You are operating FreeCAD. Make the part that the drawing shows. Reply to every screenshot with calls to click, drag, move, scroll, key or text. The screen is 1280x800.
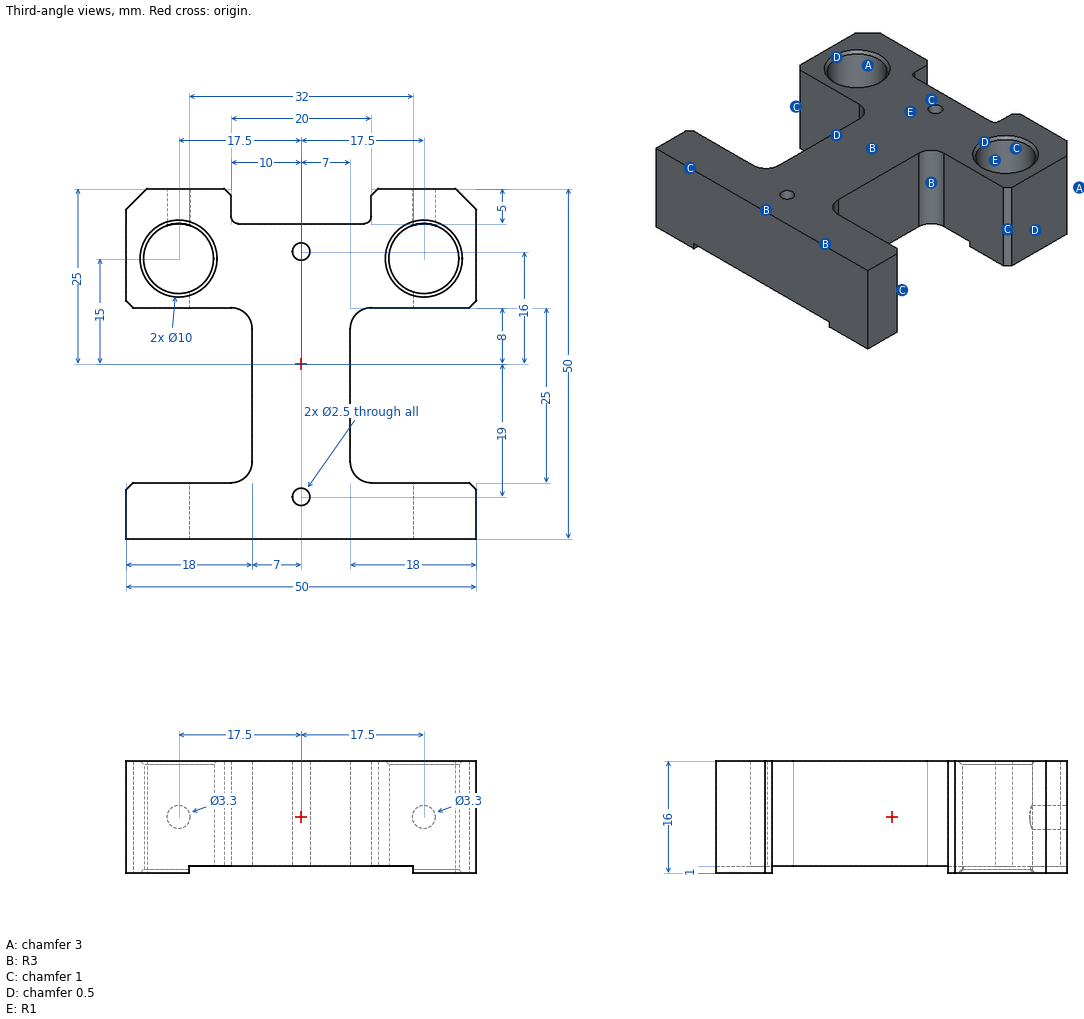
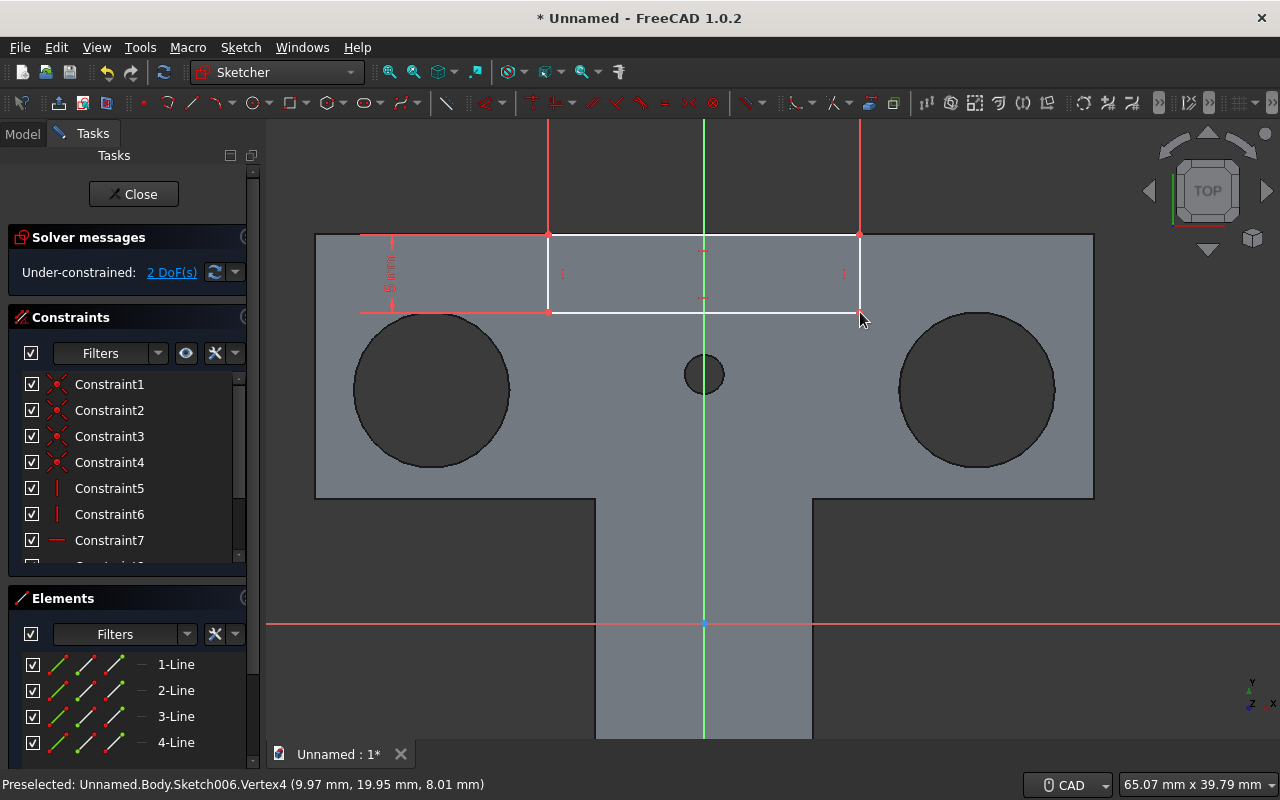
click(486, 104)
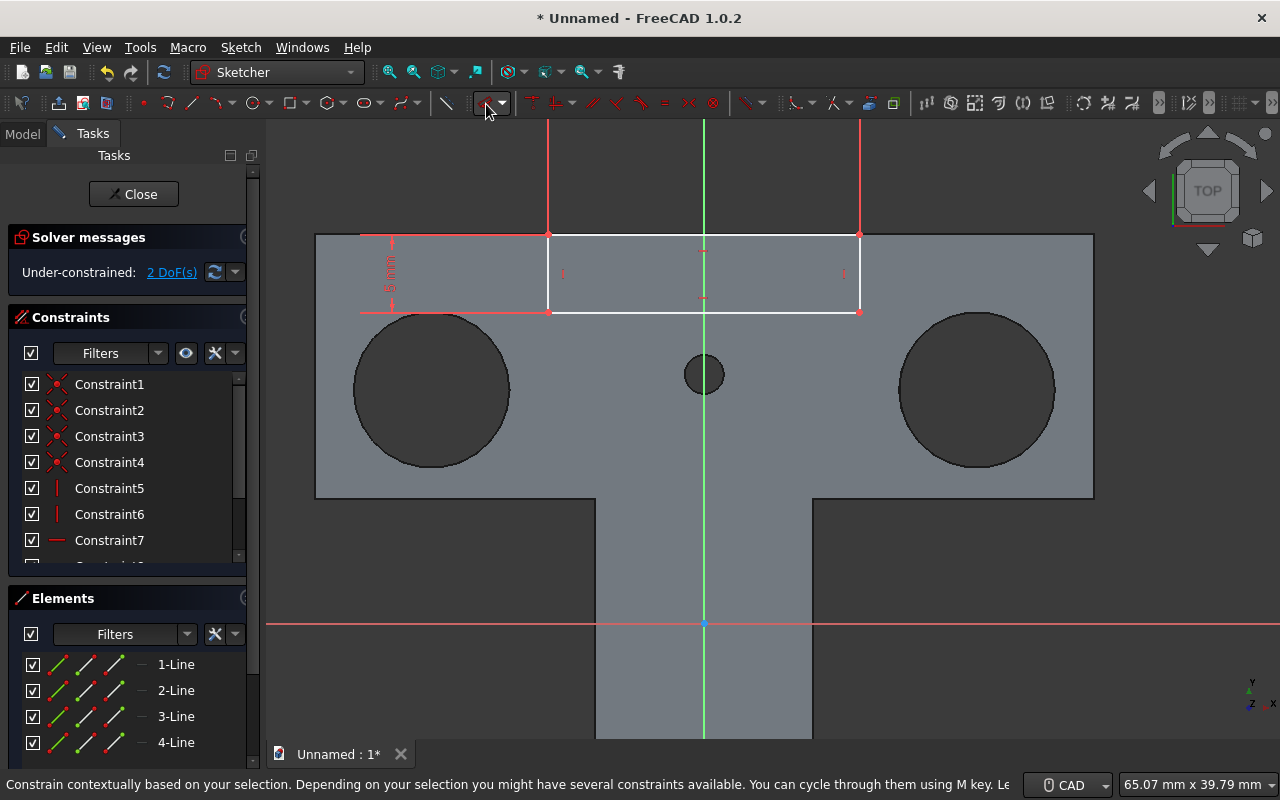
click(548, 235)
click(626, 658)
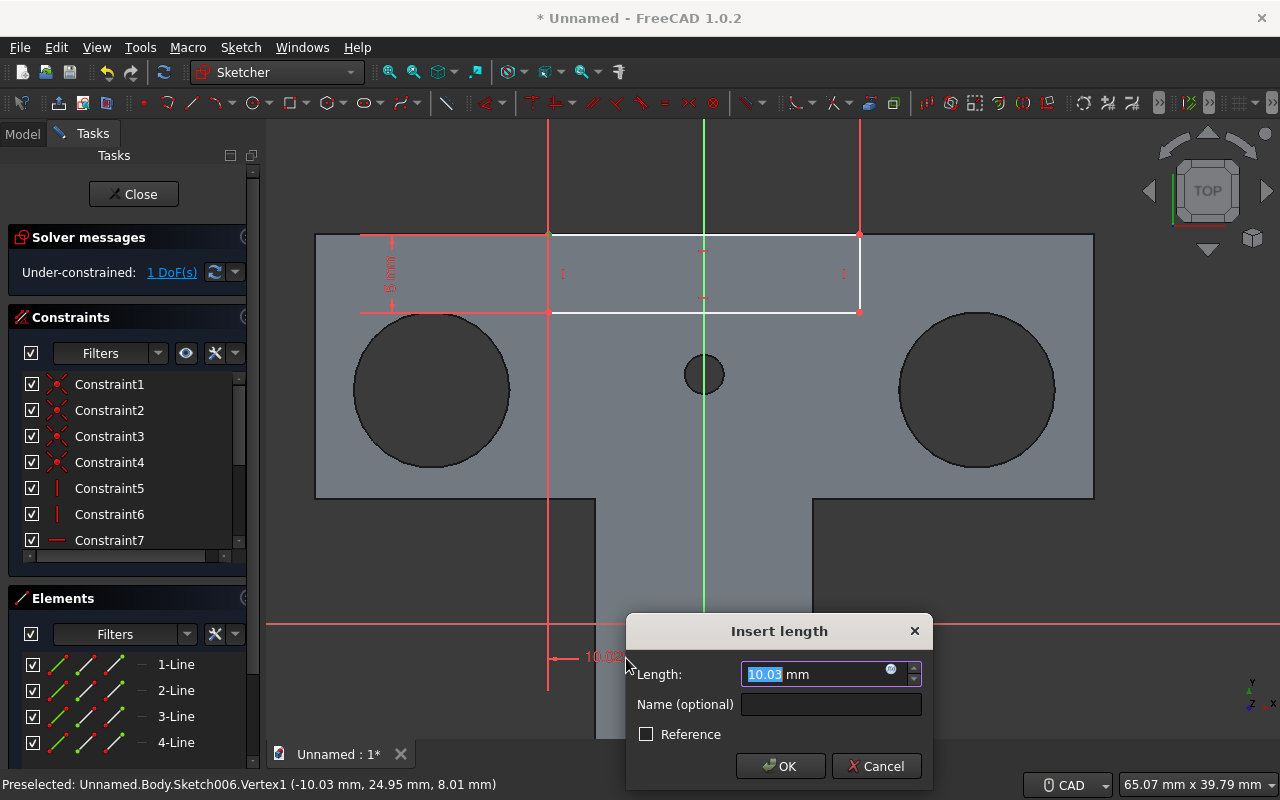
text(10)
key(Return)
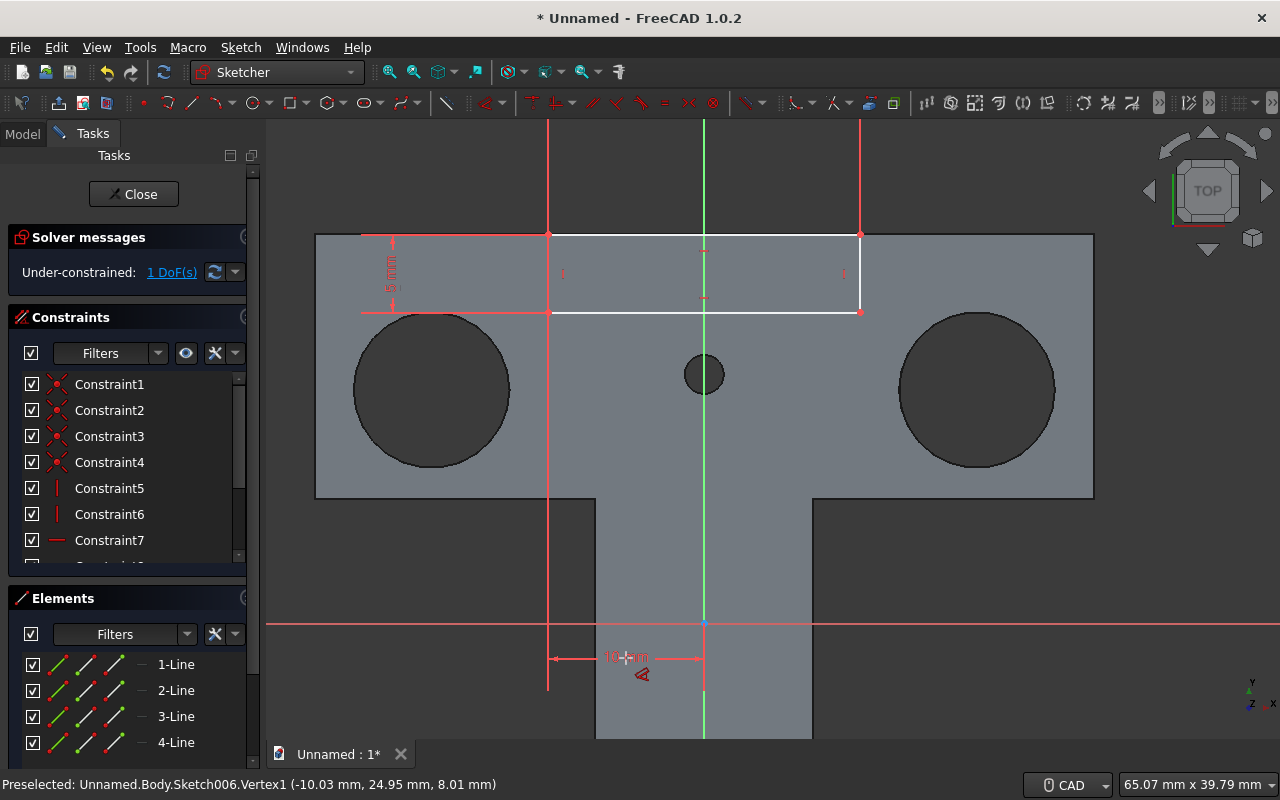
click(548, 235)
click(514, 429)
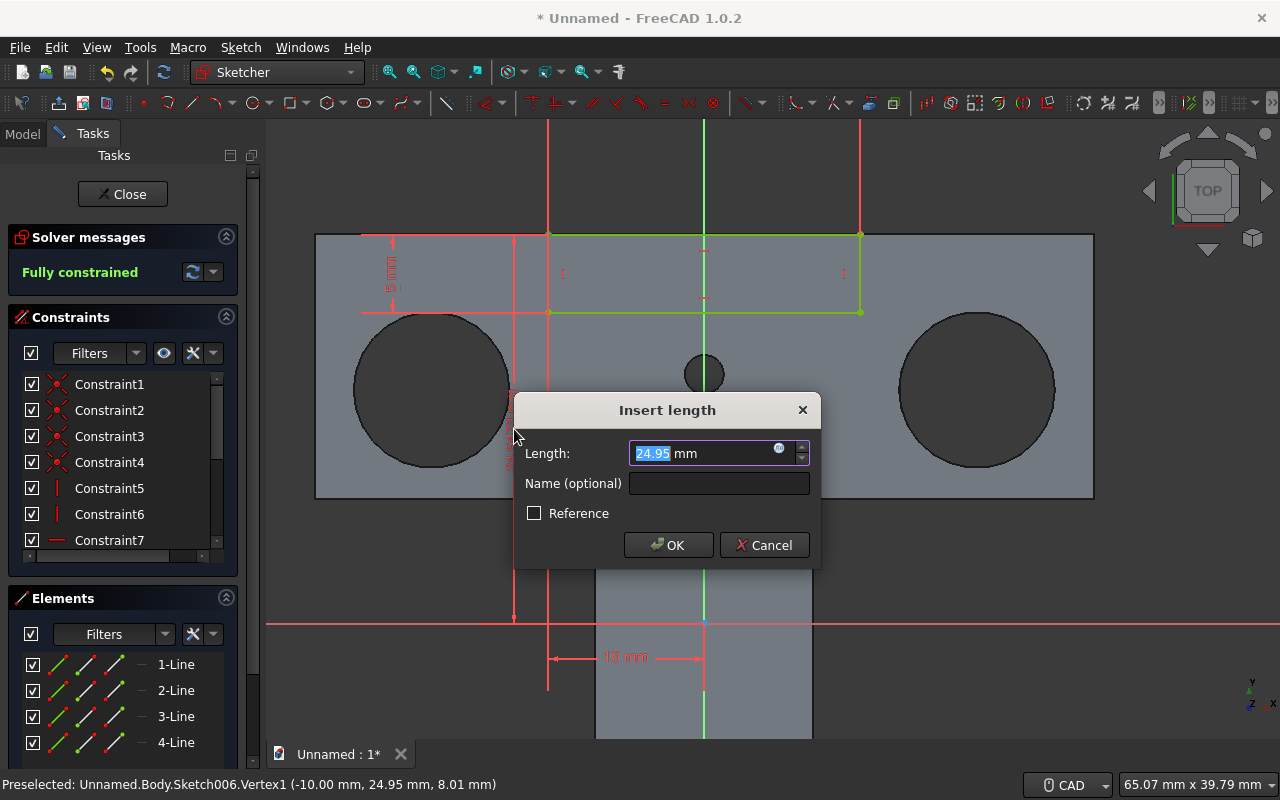
text(25)
key(Return)
key(Escape)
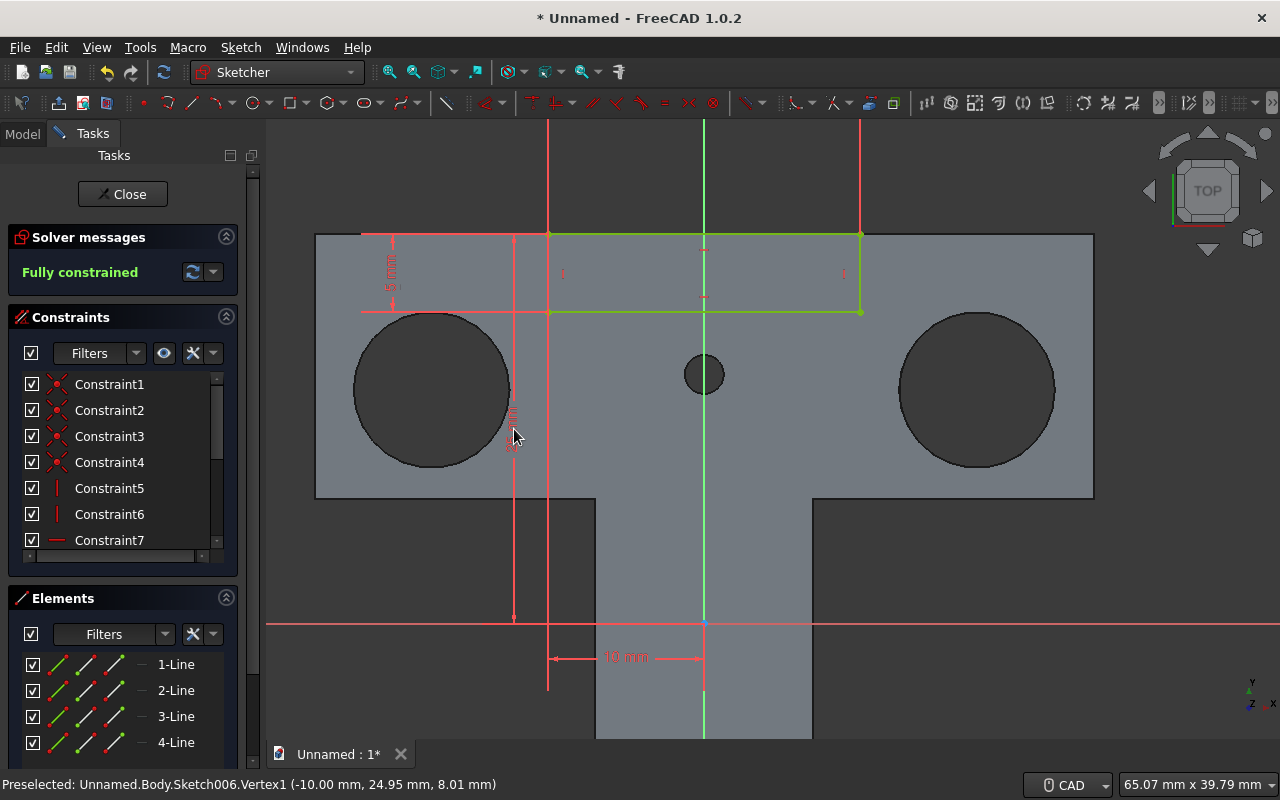
click(123, 194)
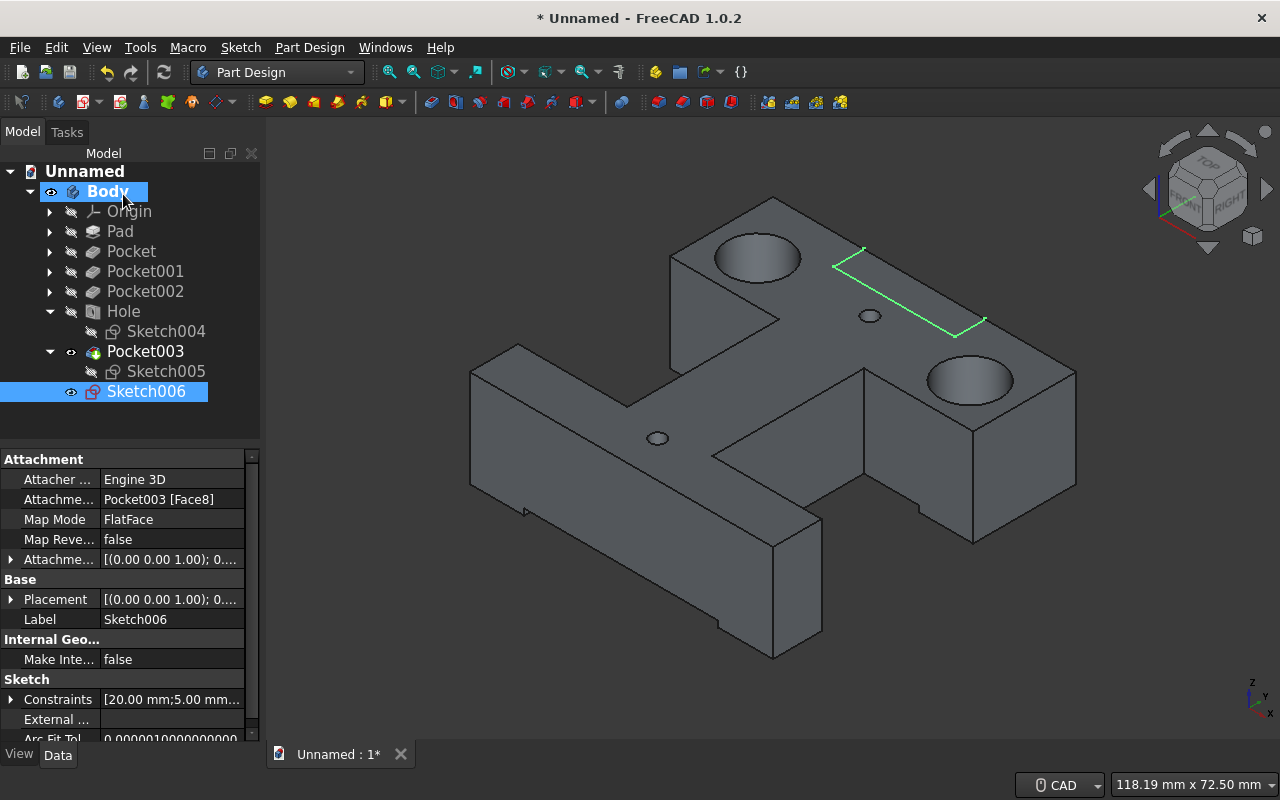
click(432, 102)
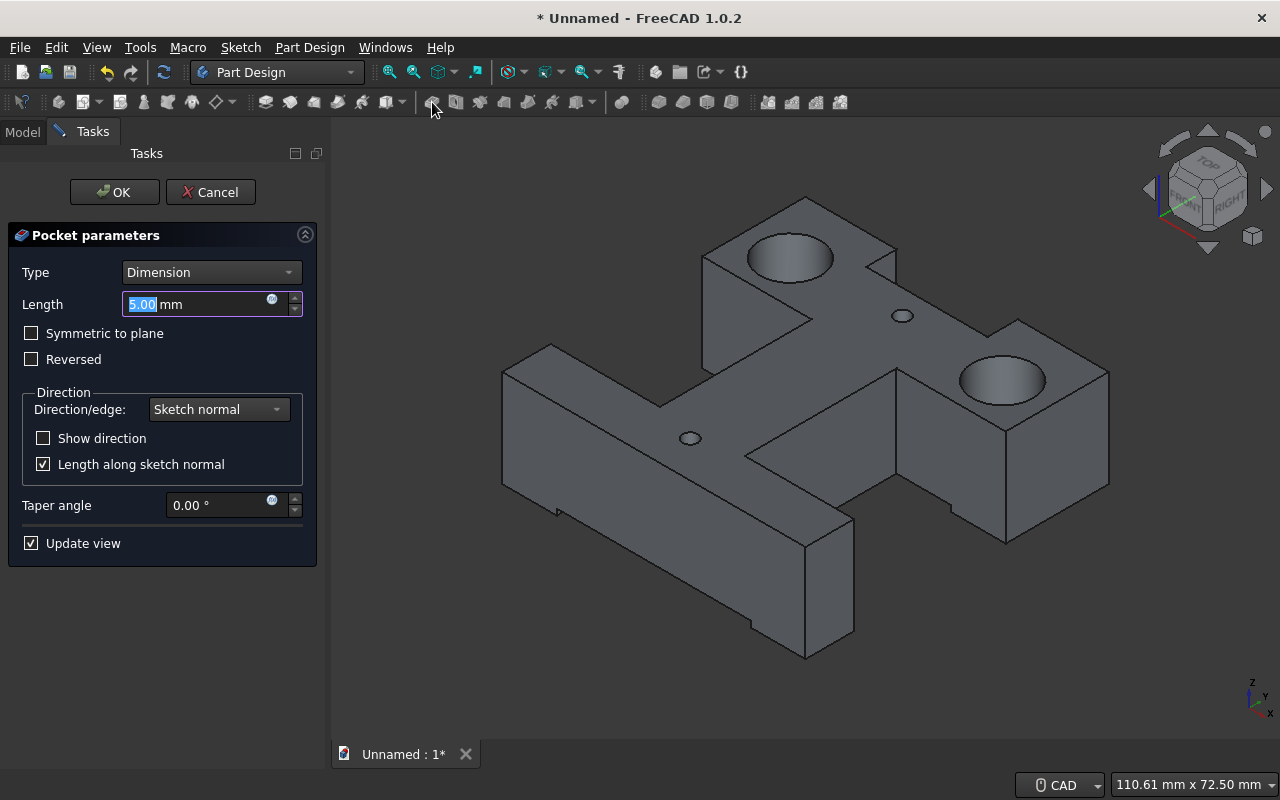
click(212, 272)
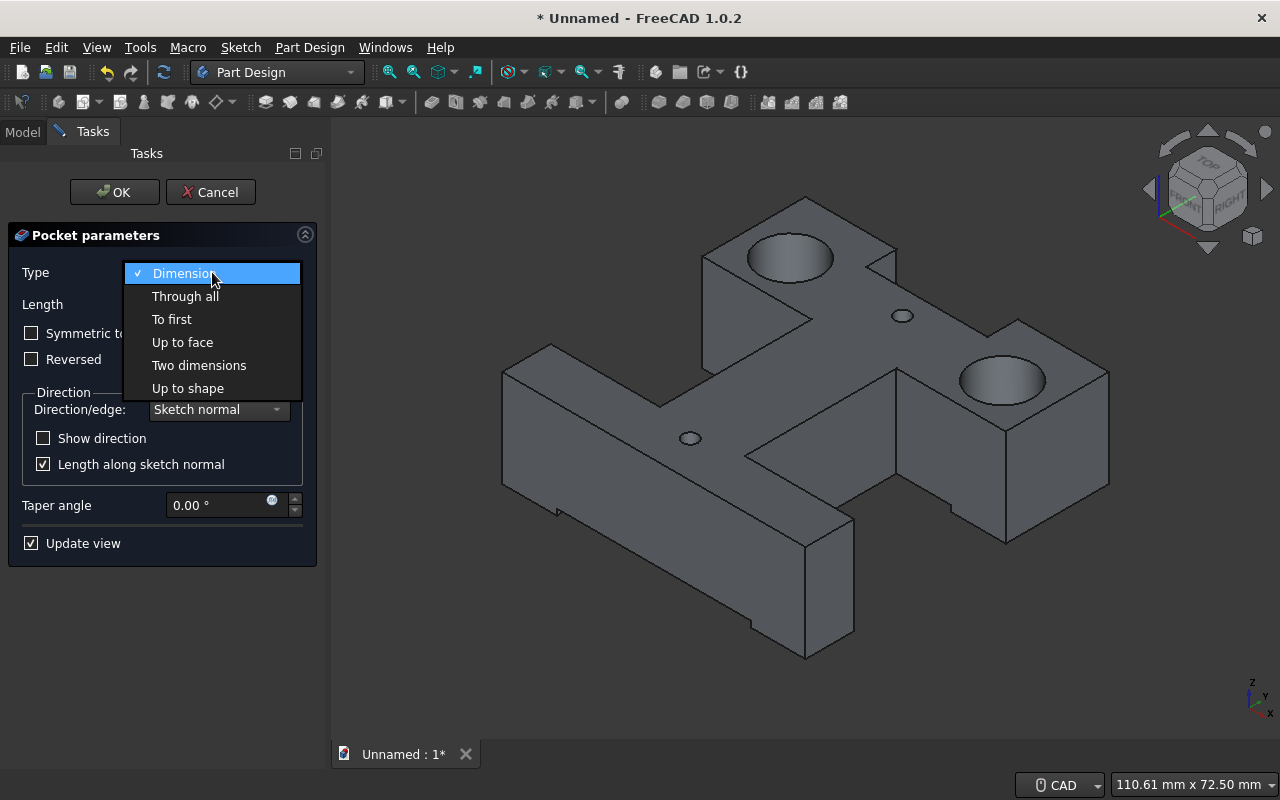
click(212, 296)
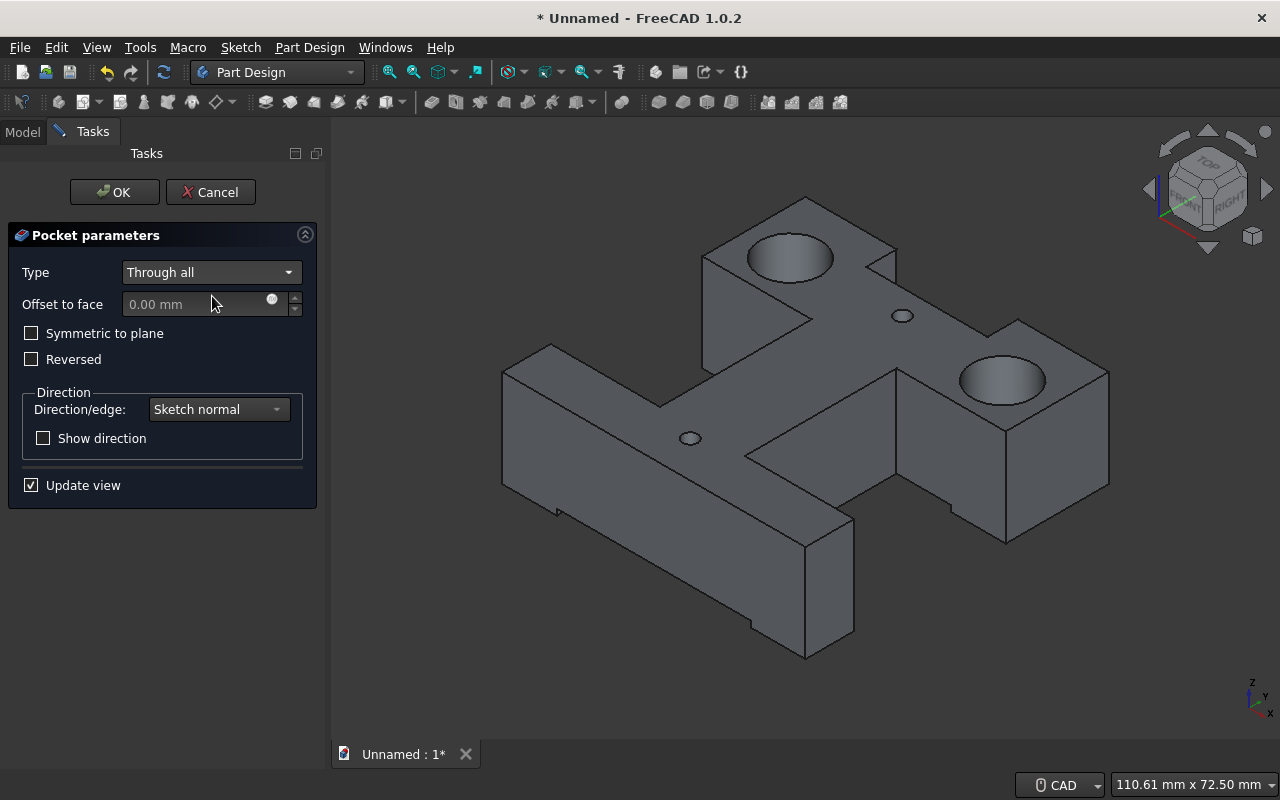
click(115, 192)